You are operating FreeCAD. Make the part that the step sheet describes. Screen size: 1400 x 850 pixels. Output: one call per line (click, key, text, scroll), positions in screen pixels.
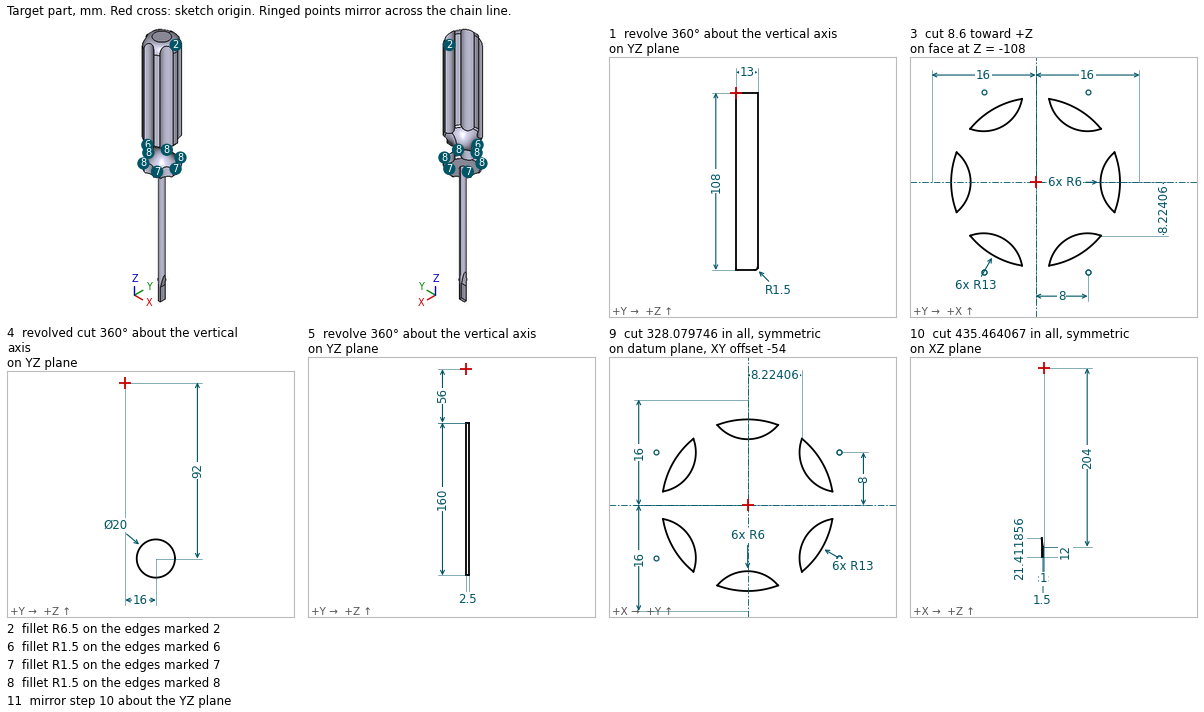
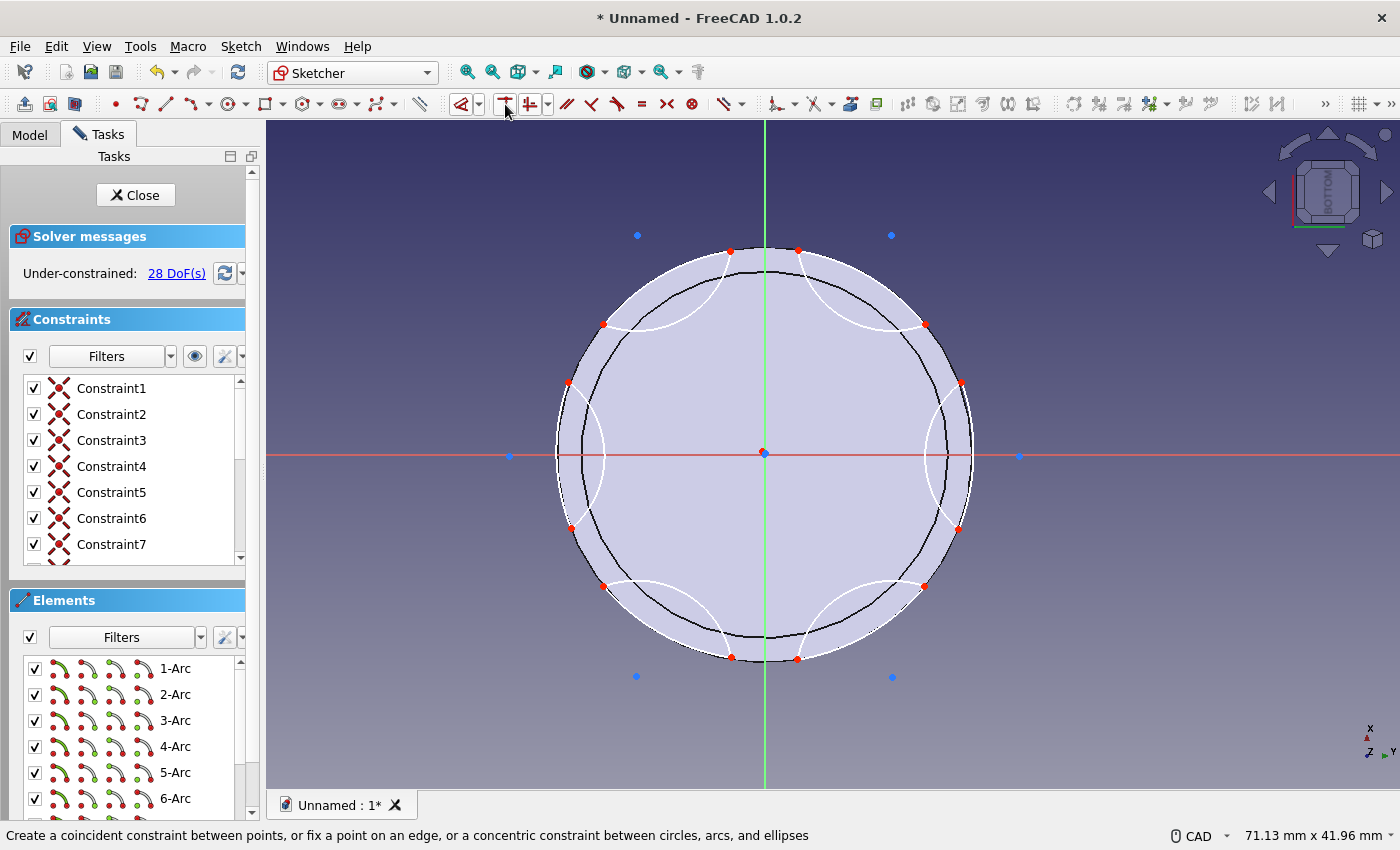
click(971, 486)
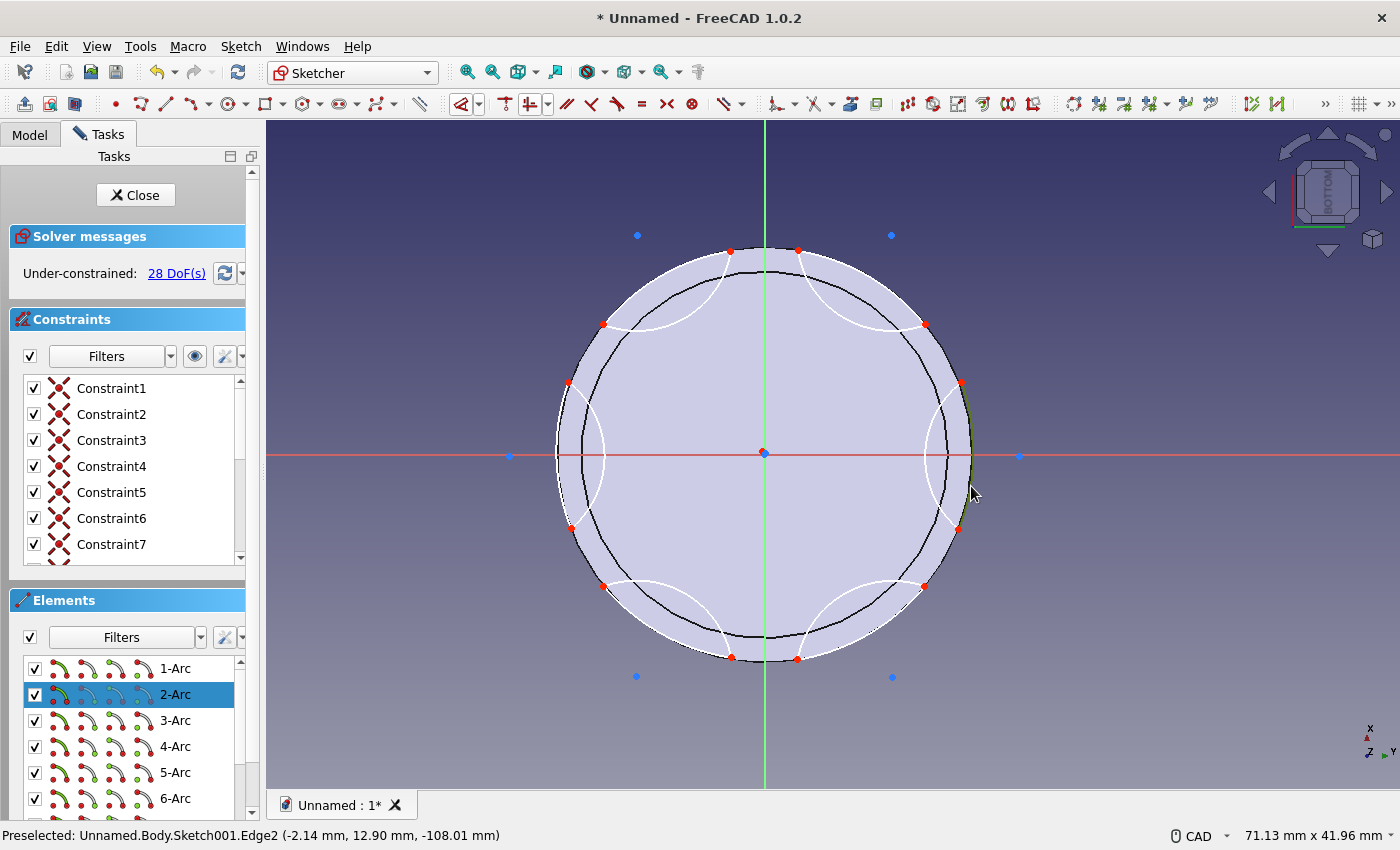
click(893, 293)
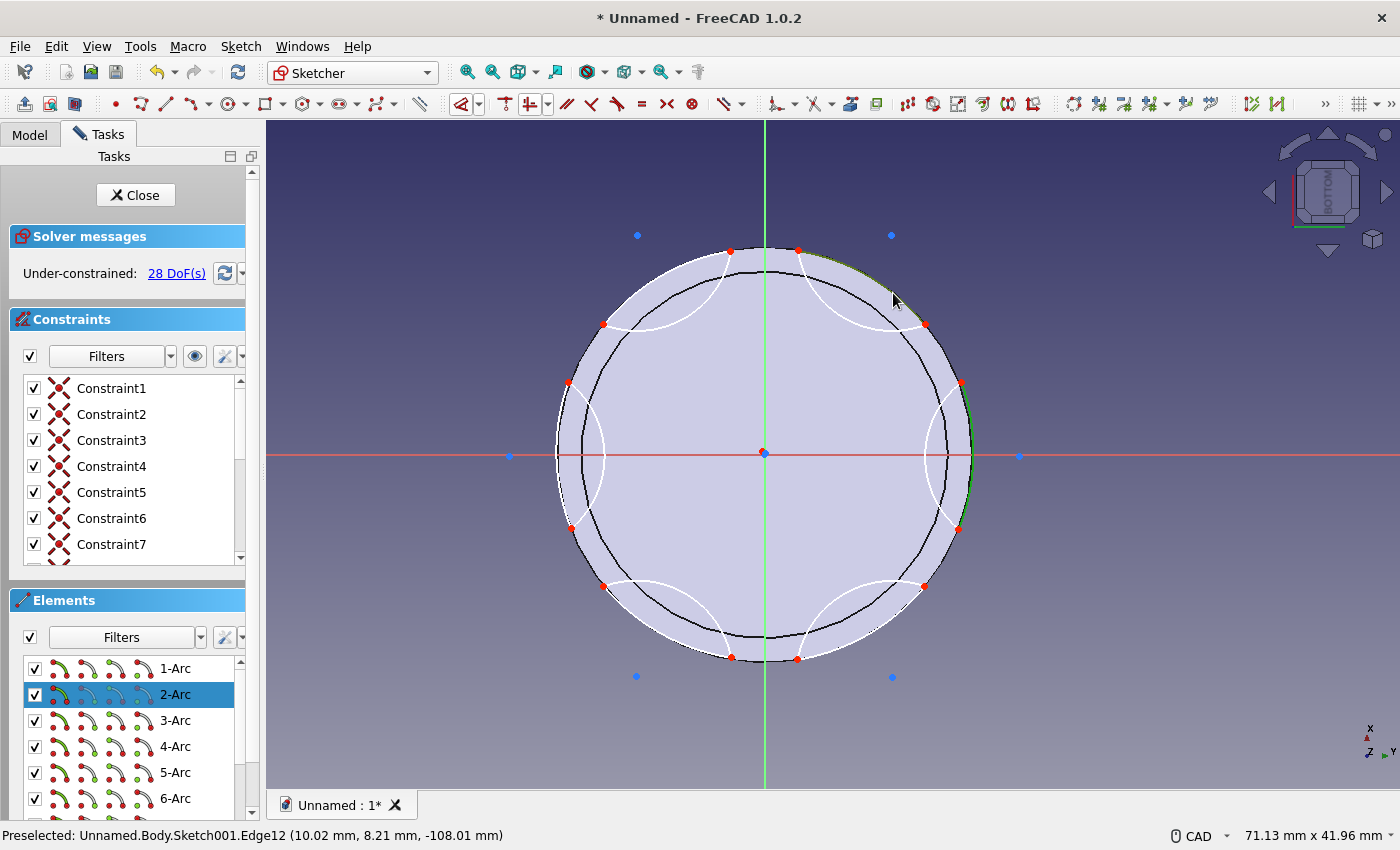
key(c)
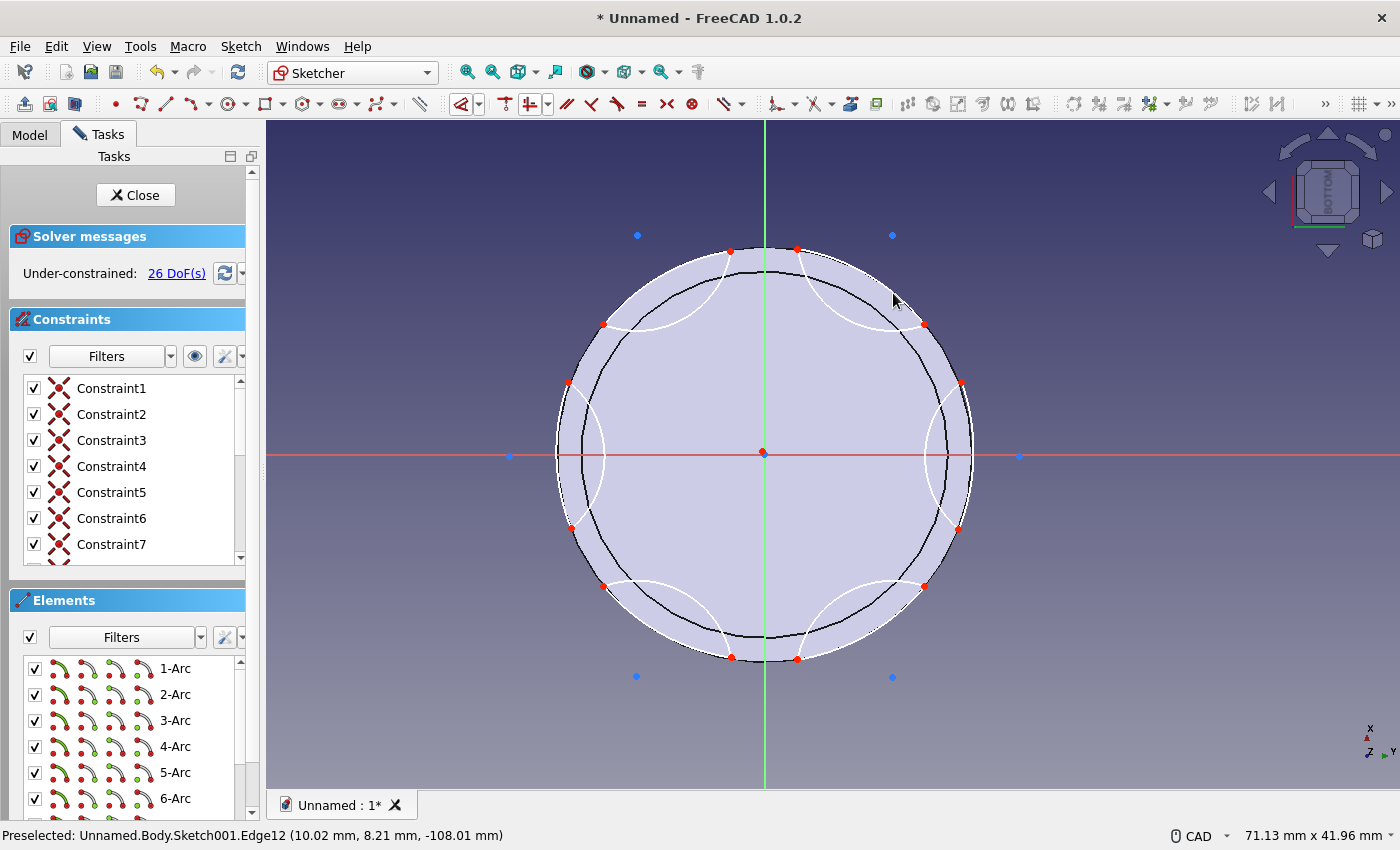
drag(753, 442, 775, 465)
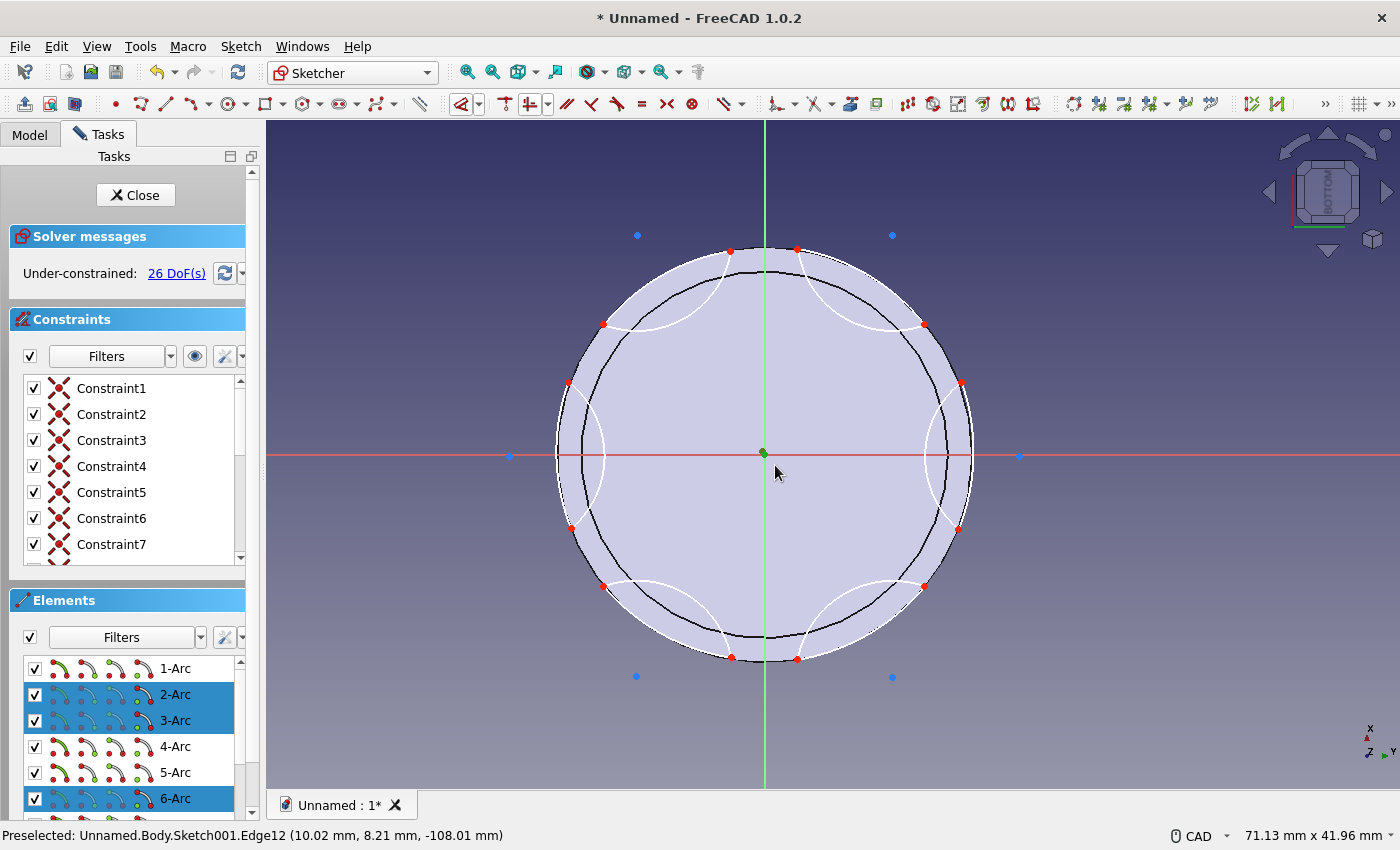
key(c)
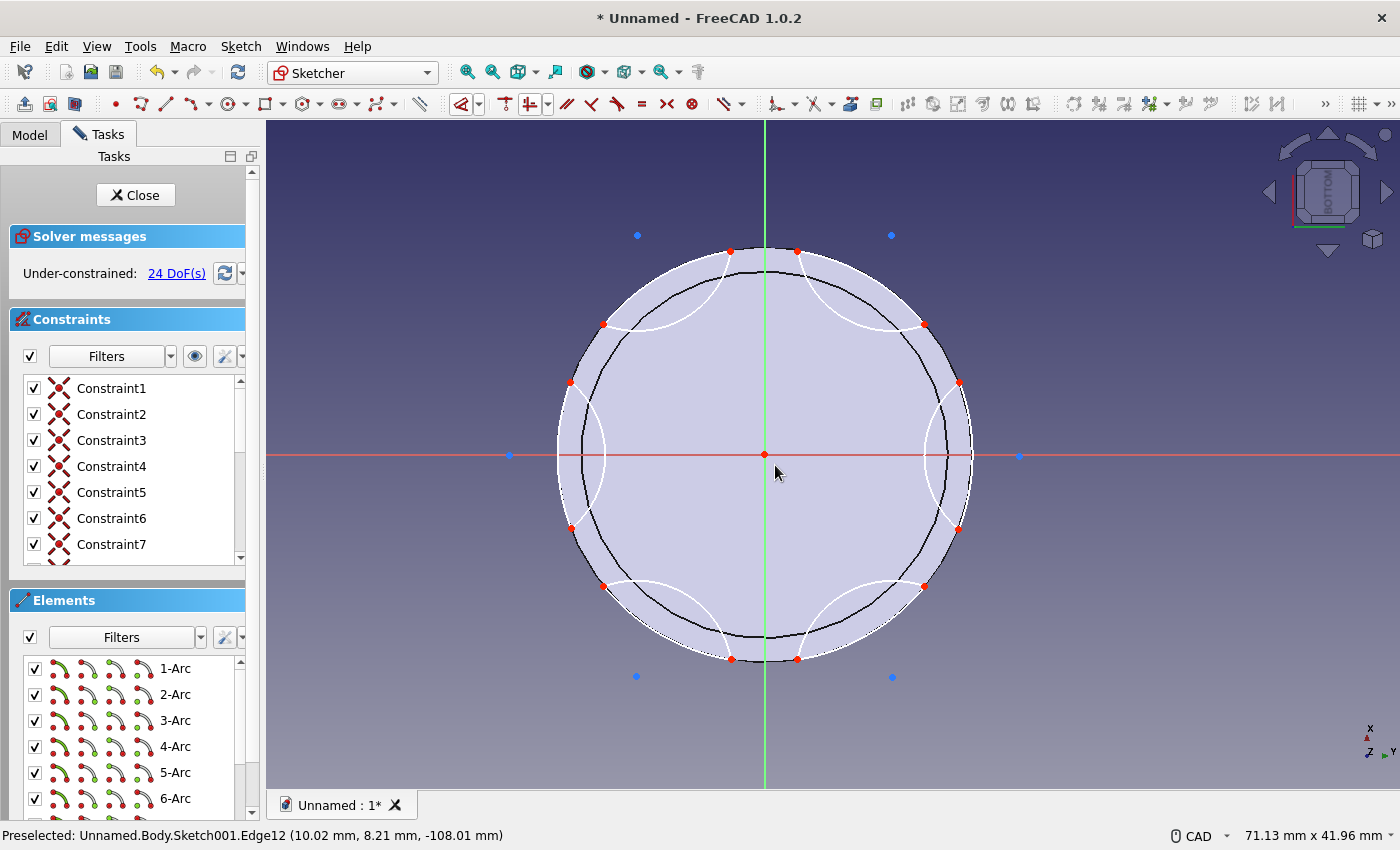
click(970, 486)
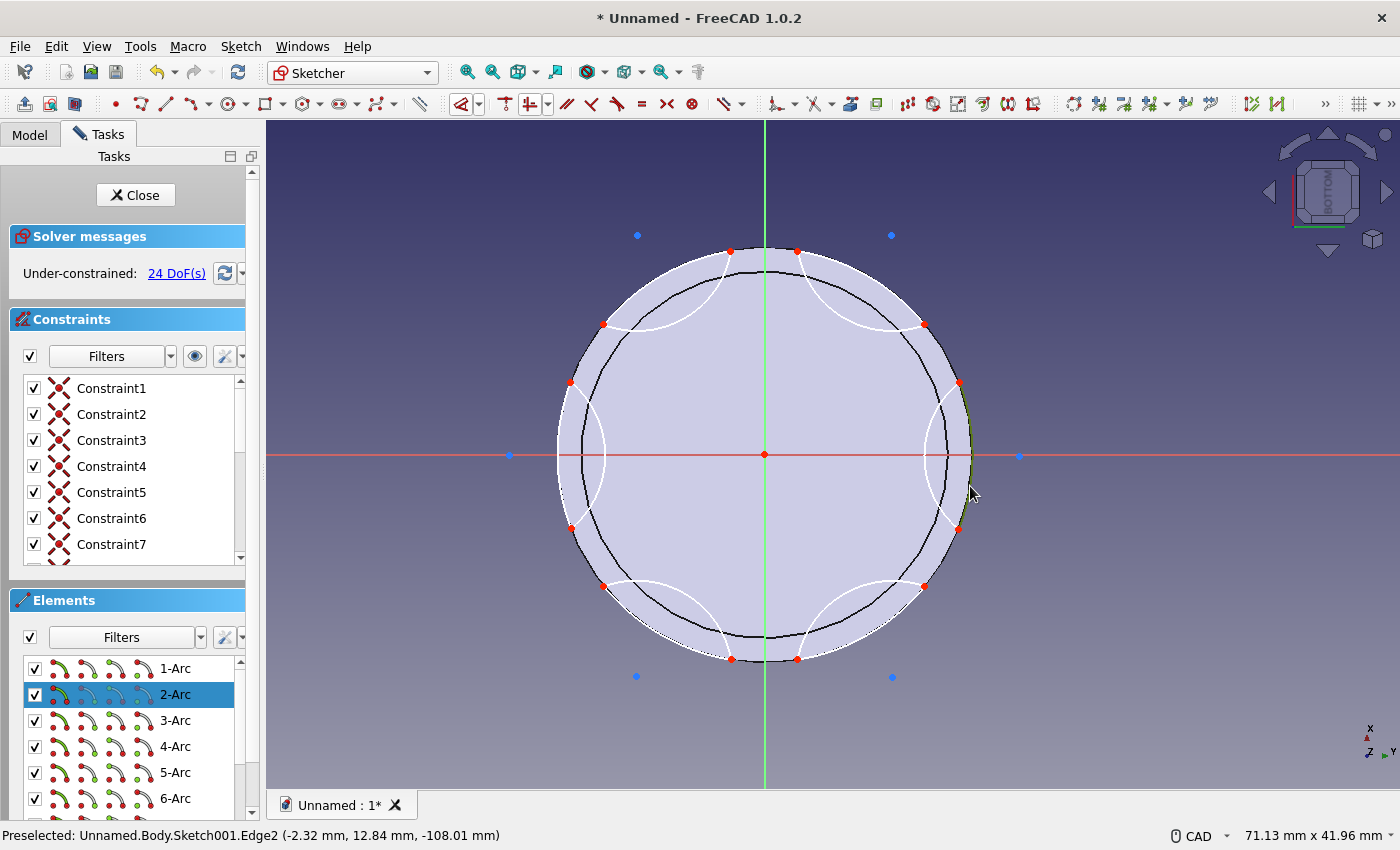
click(841, 648)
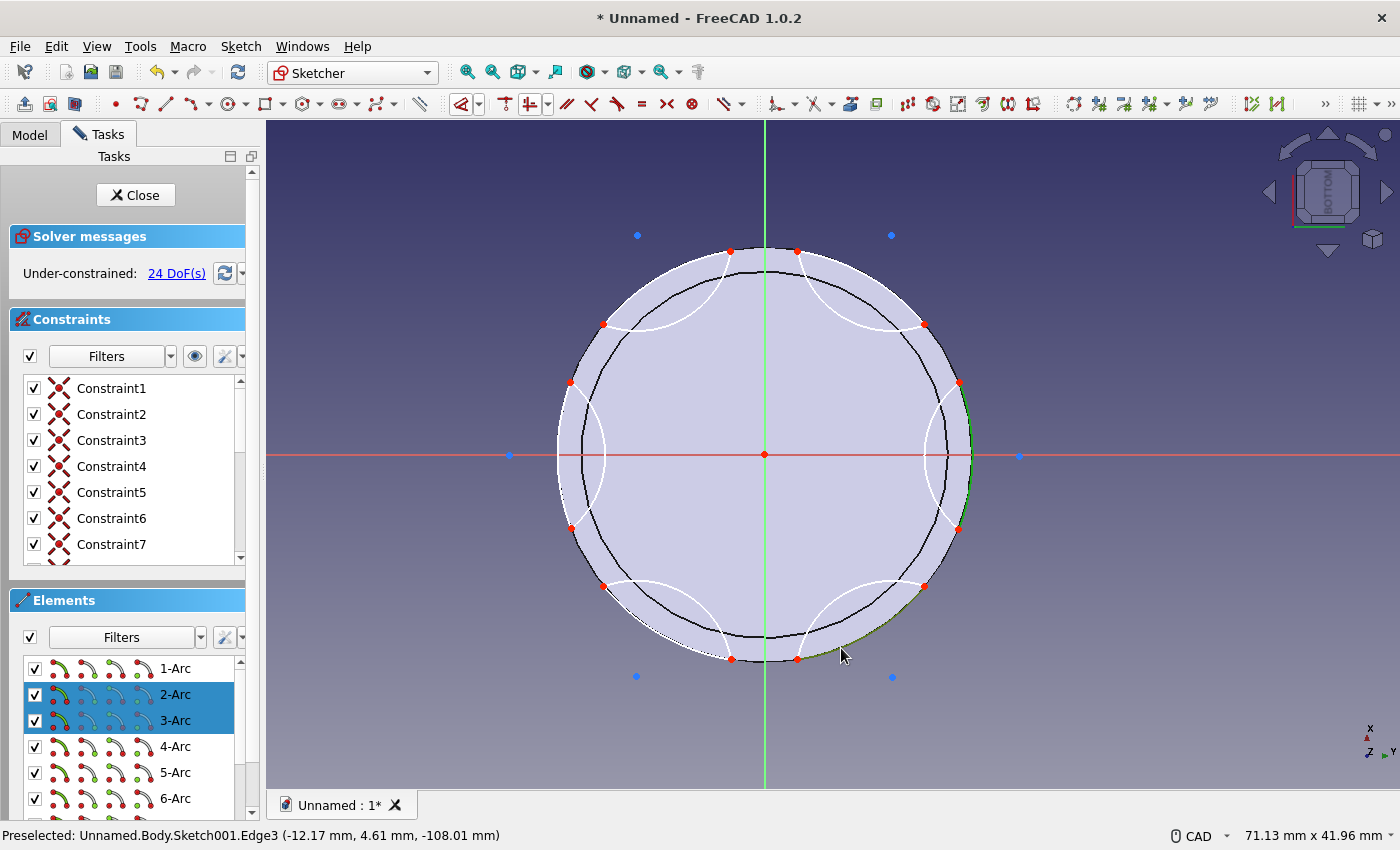
click(636, 618)